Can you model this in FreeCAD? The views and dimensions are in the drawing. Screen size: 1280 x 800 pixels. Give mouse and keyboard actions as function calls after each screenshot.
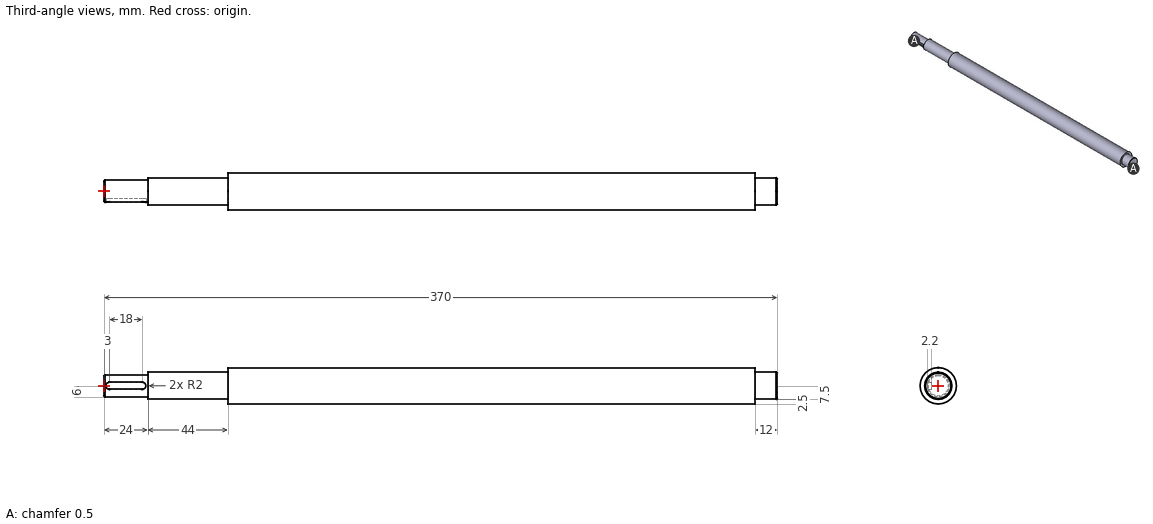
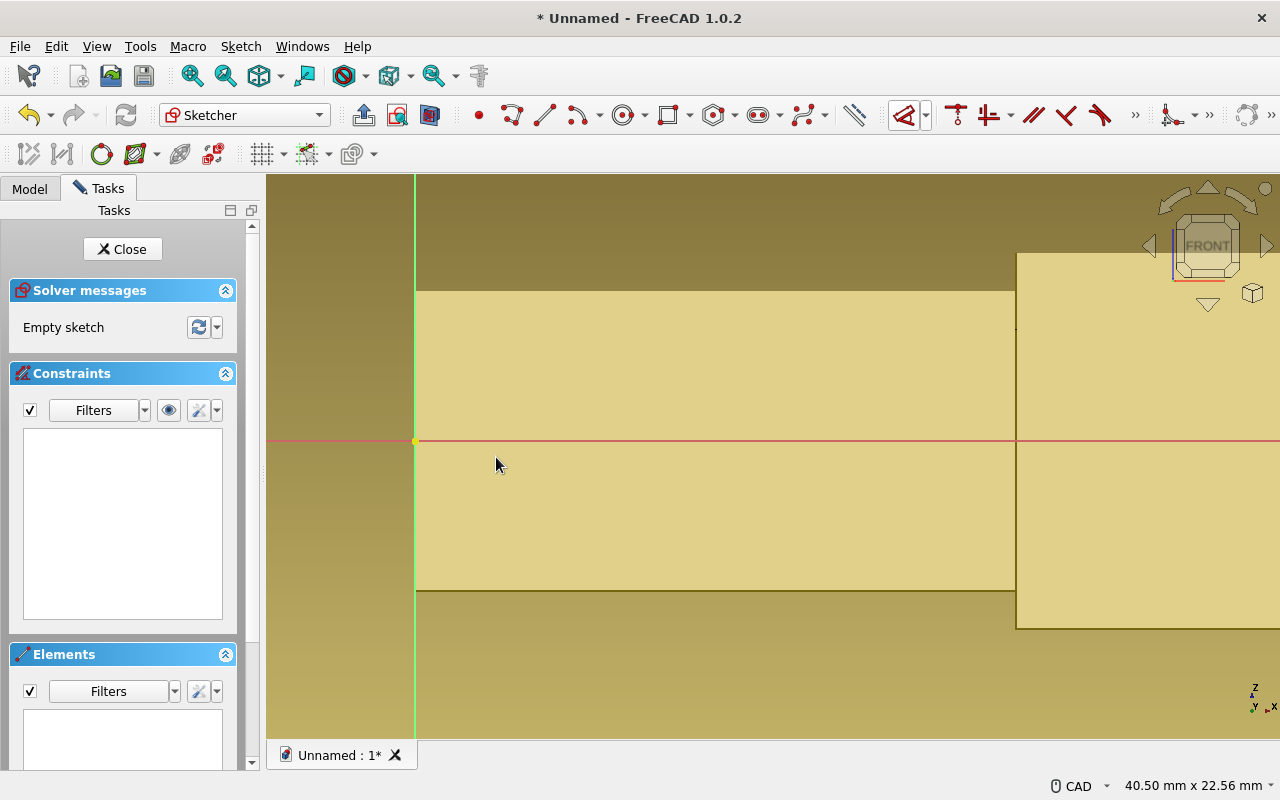
click(758, 116)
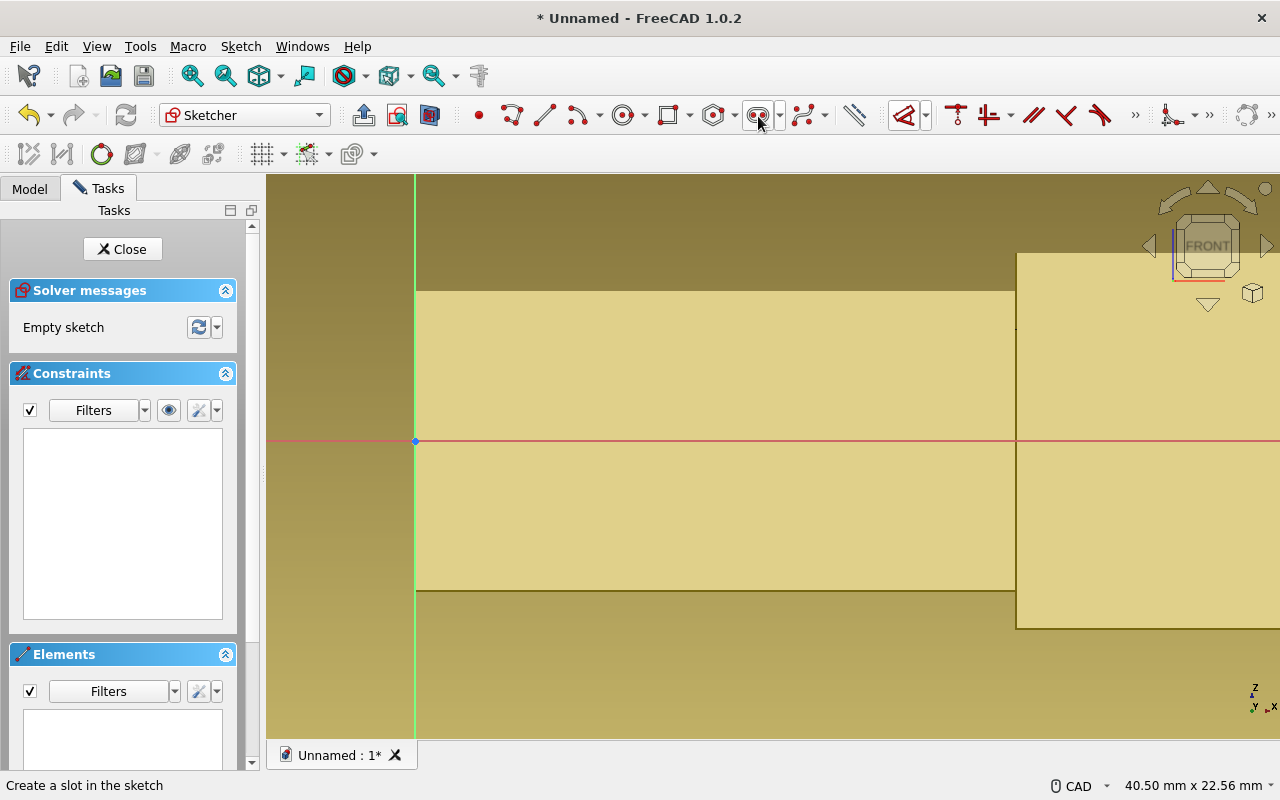
click(491, 441)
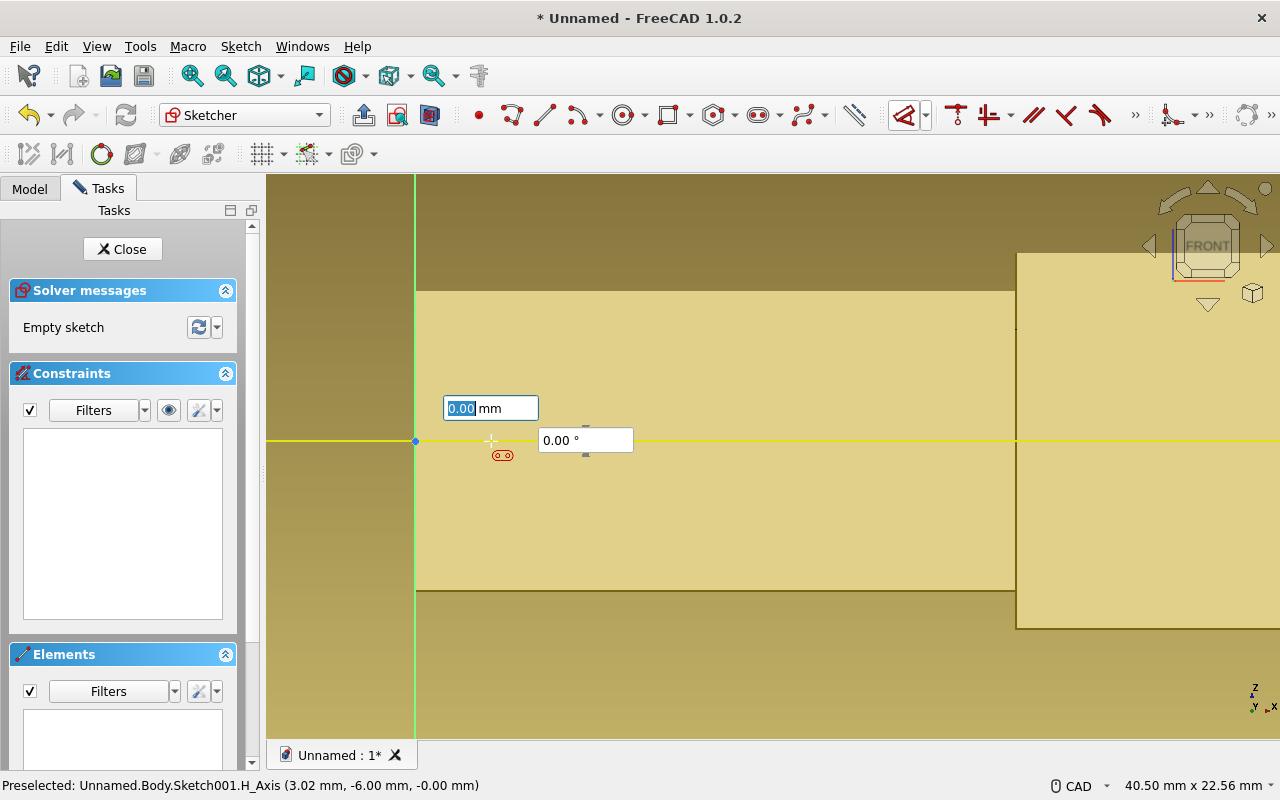
click(941, 432)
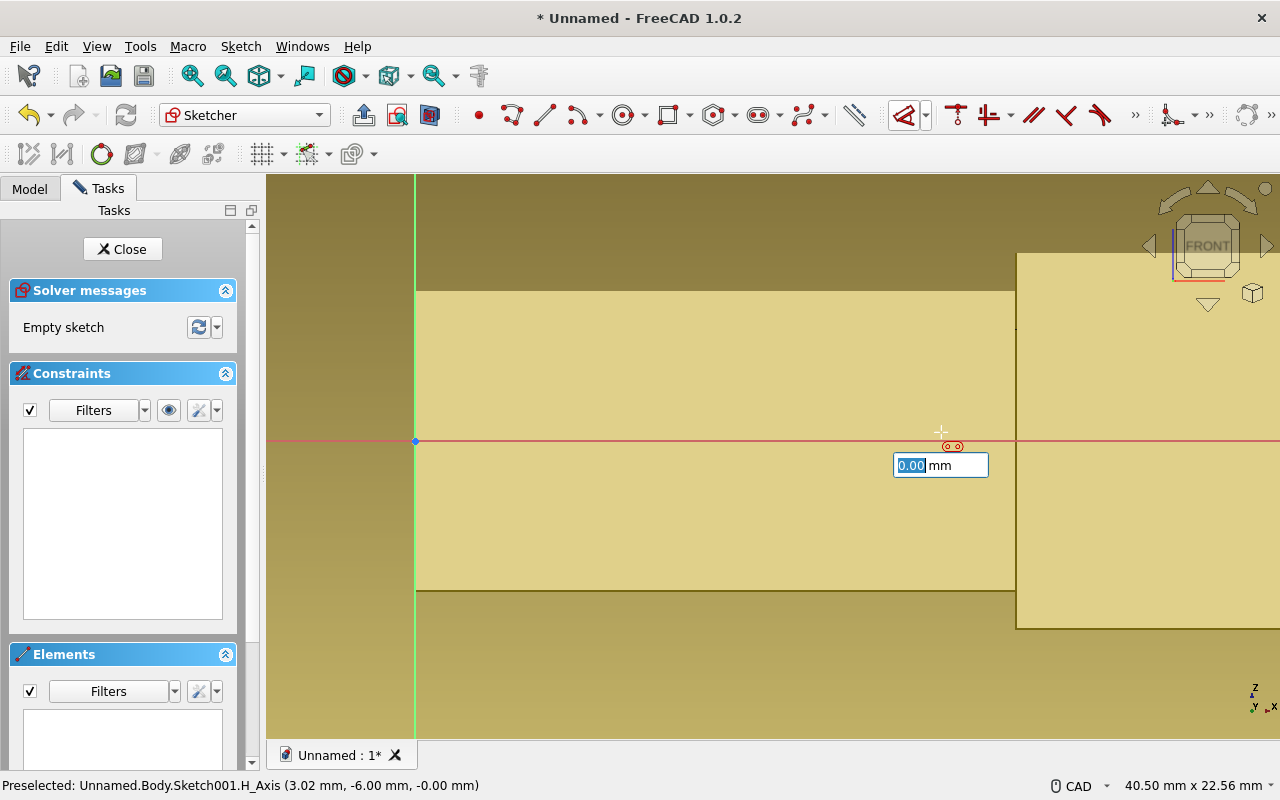
click(716, 491)
key(Escape)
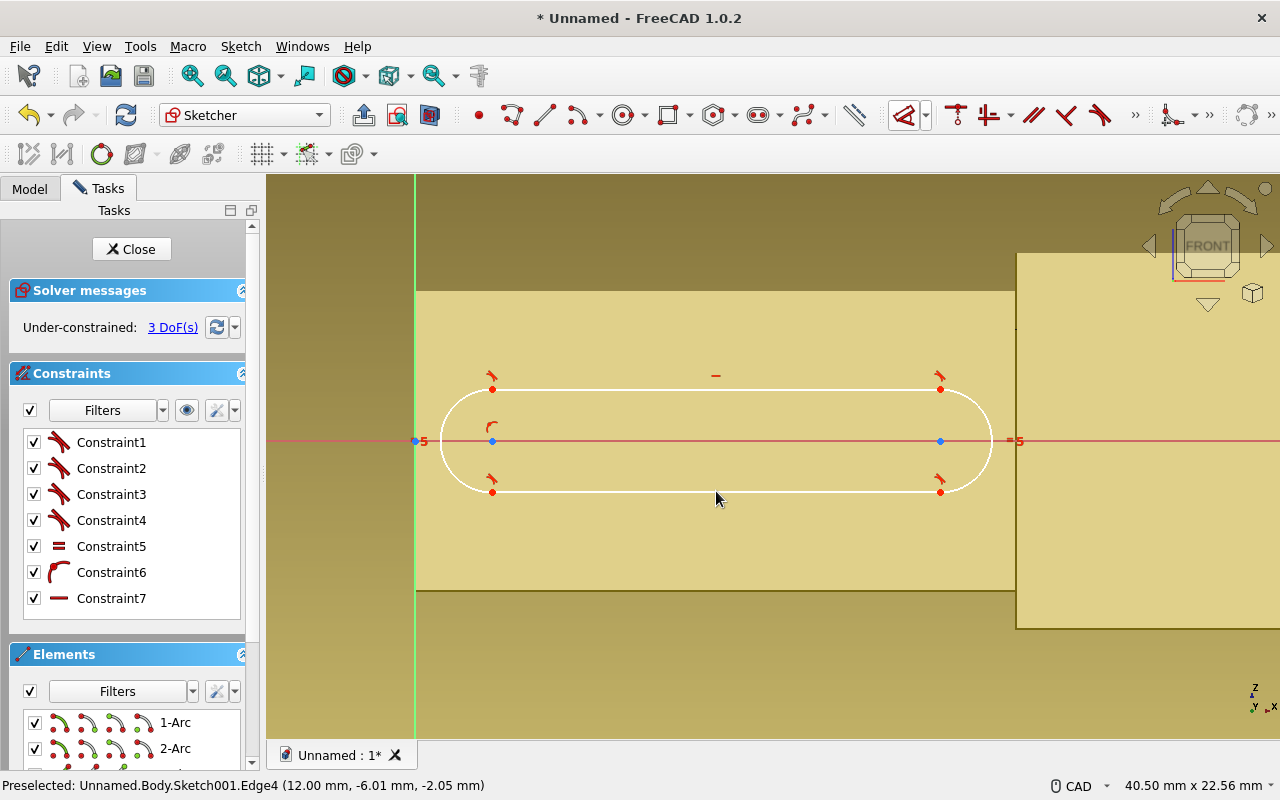
key(d)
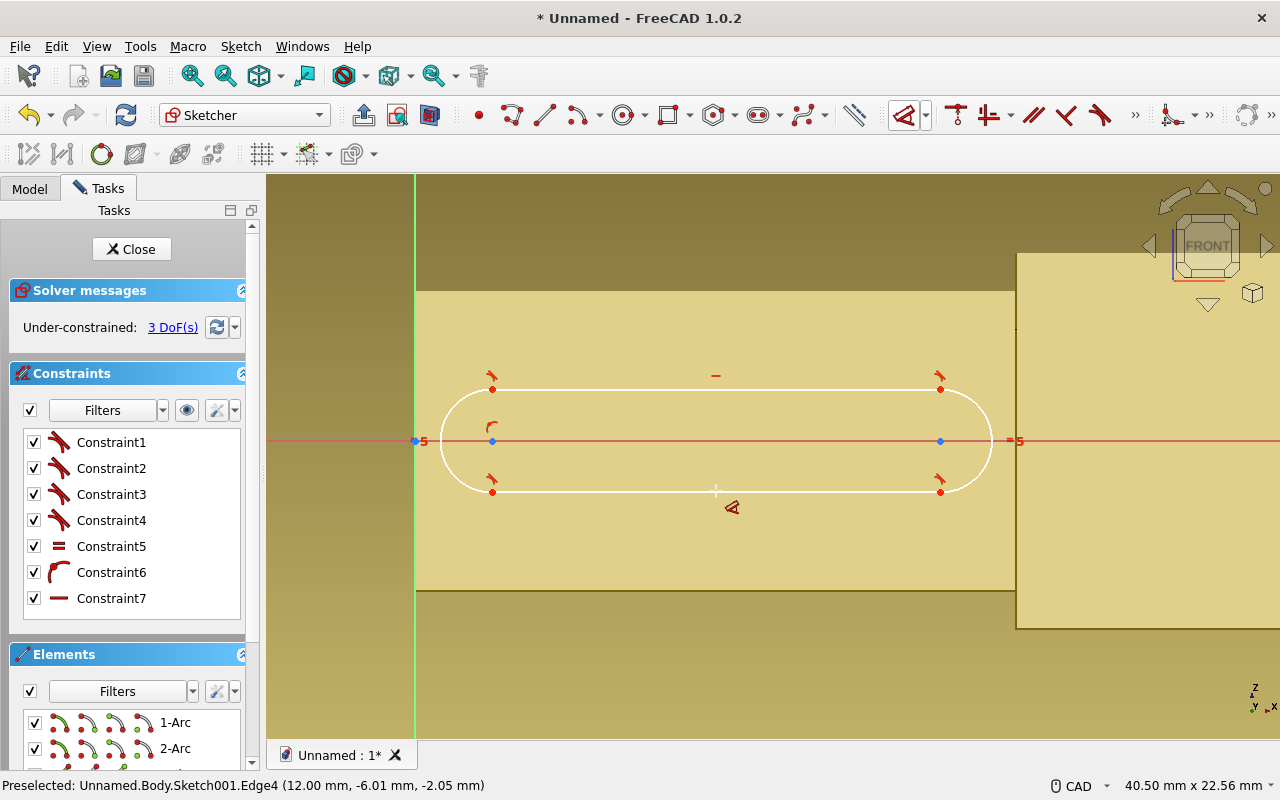
click(450, 411)
click(456, 366)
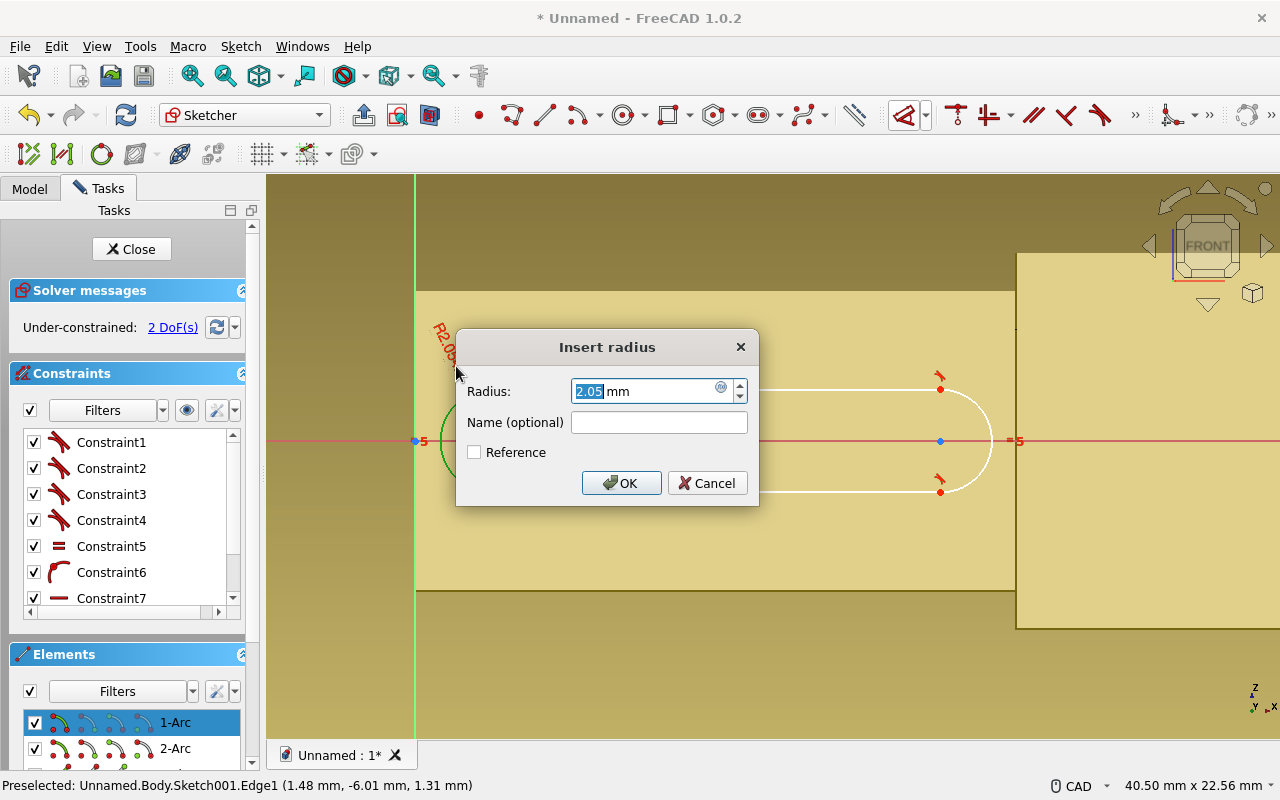
text(2)
key(Return)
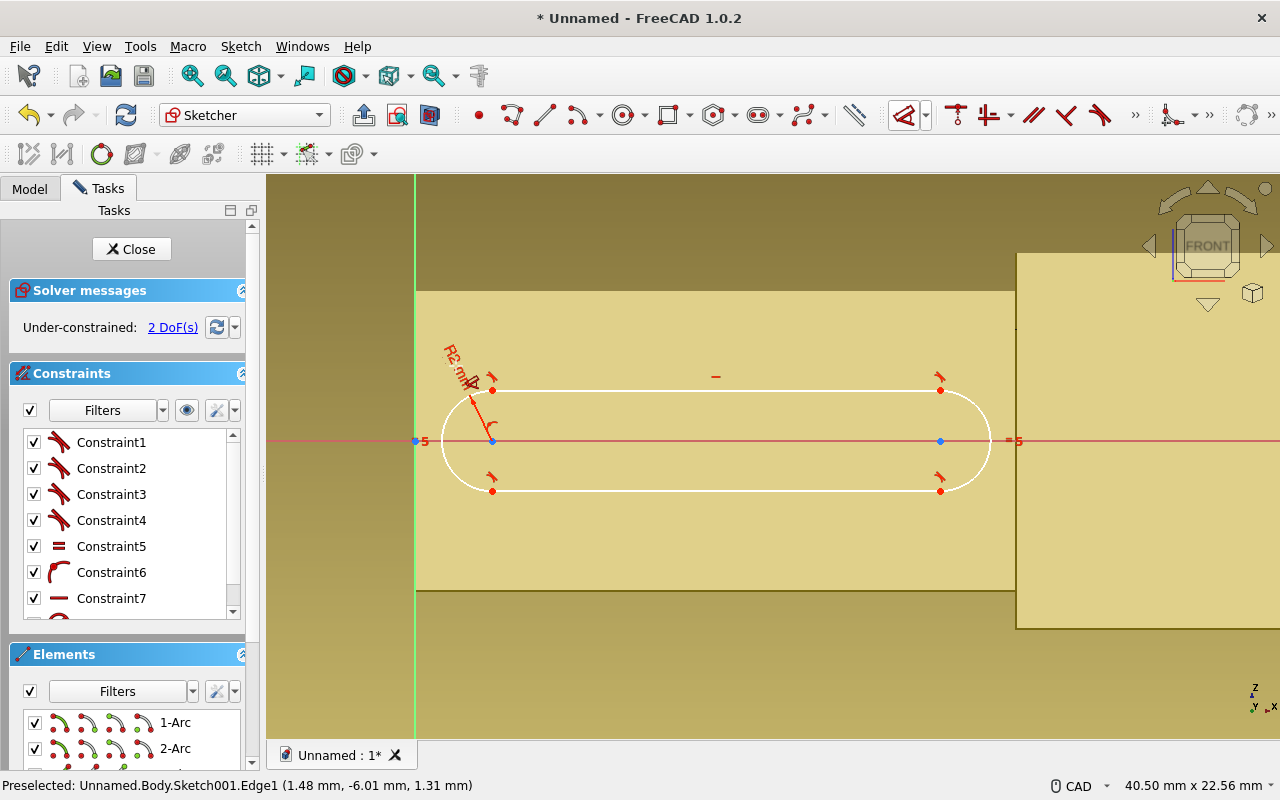
click(627, 391)
click(716, 357)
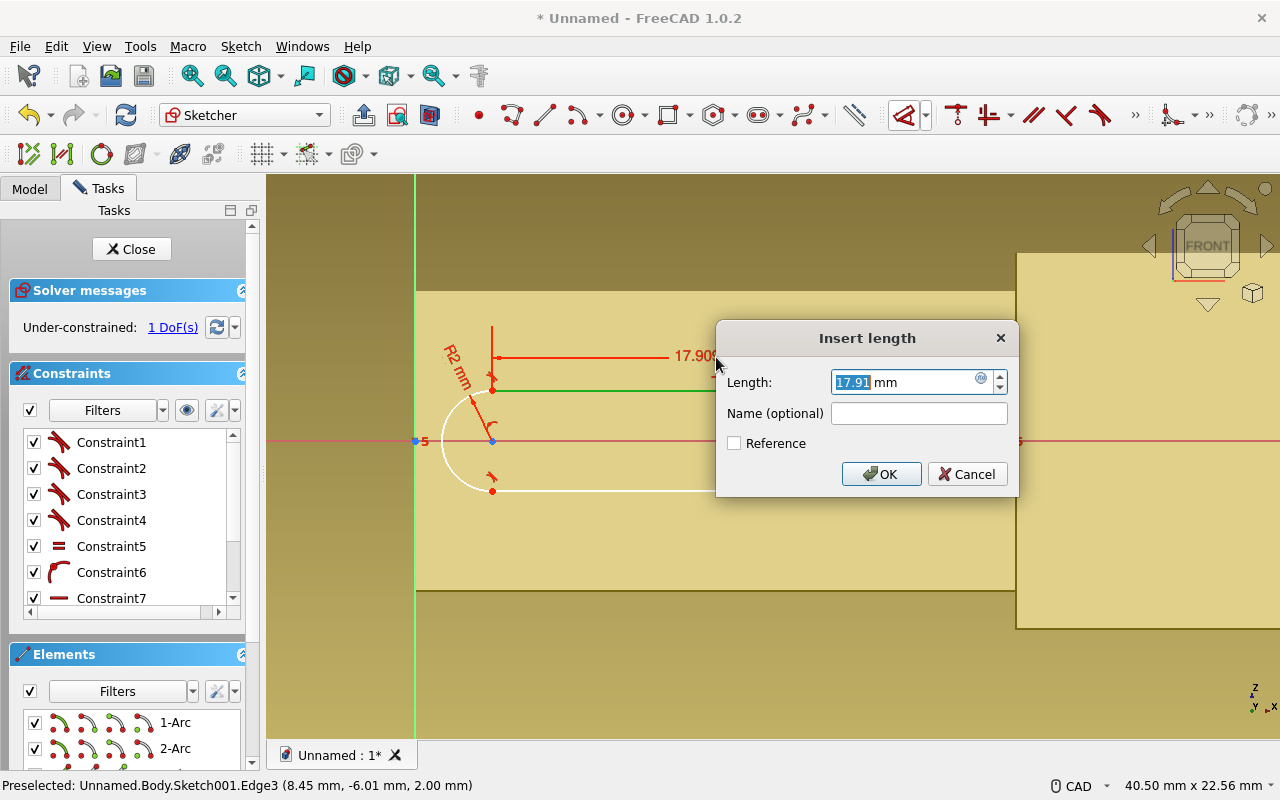
text(18)
key(Return)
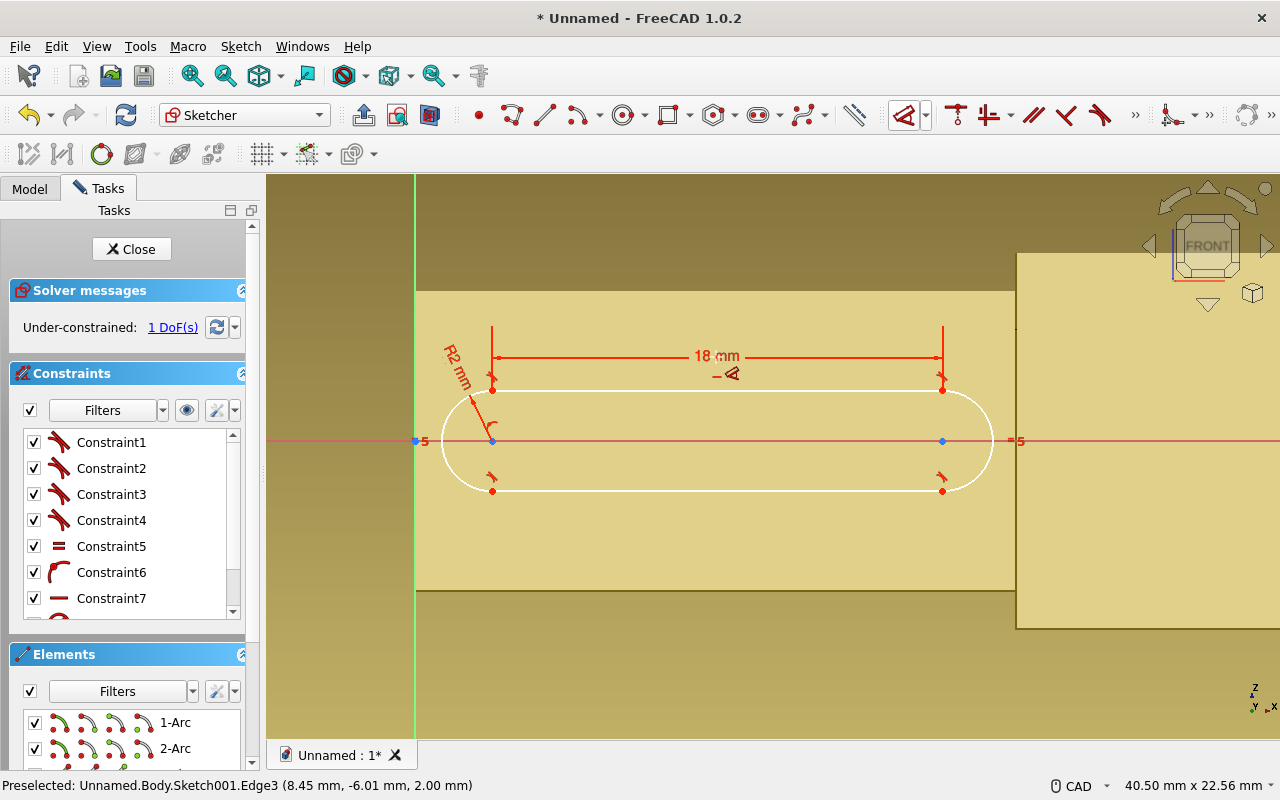
click(492, 391)
click(436, 475)